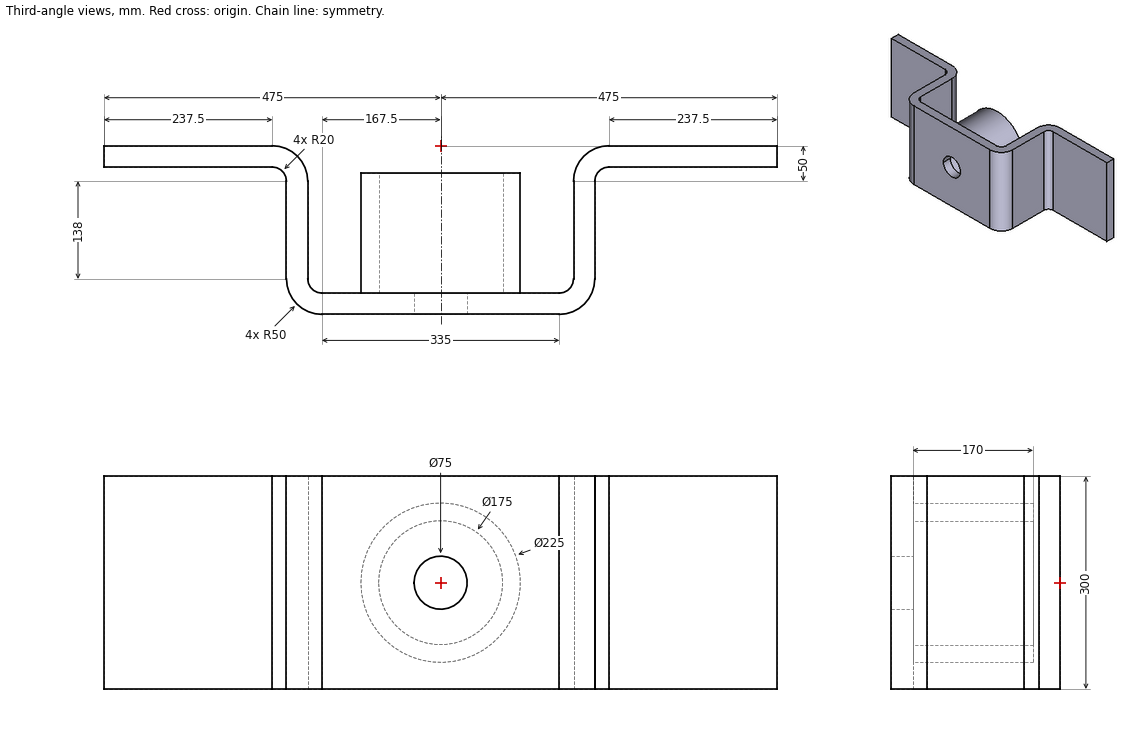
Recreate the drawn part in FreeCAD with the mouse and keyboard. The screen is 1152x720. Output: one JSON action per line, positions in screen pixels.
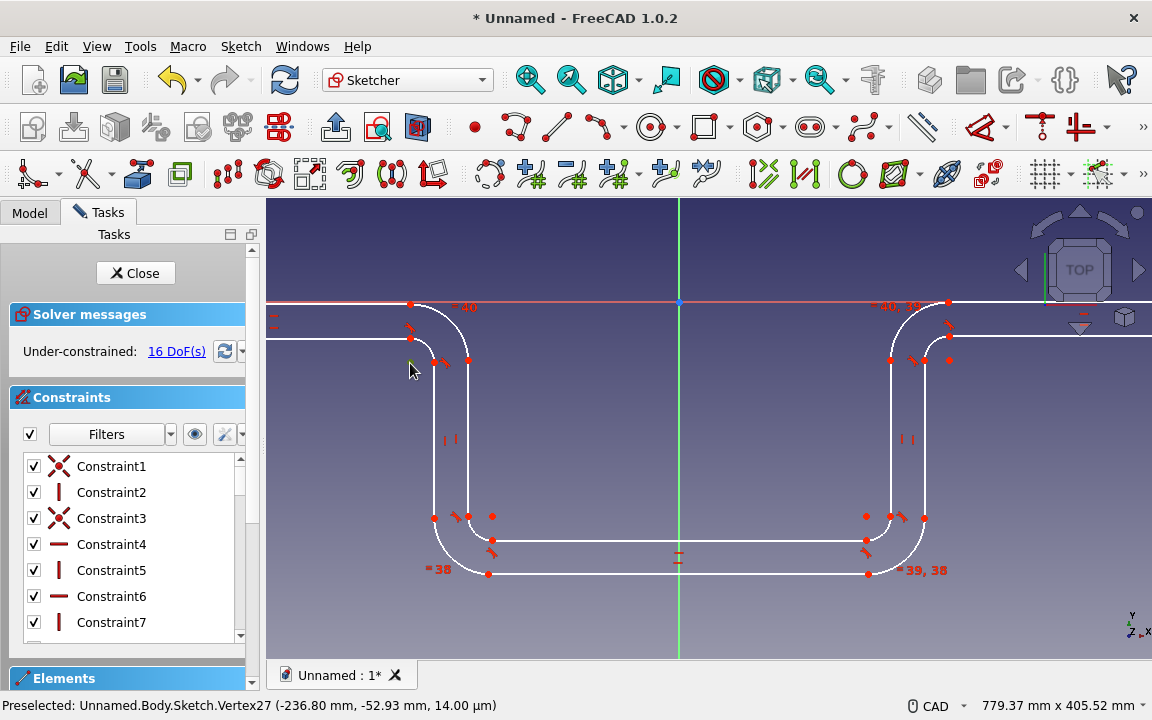
{"action": "left_click", "coordinate": [949, 361]}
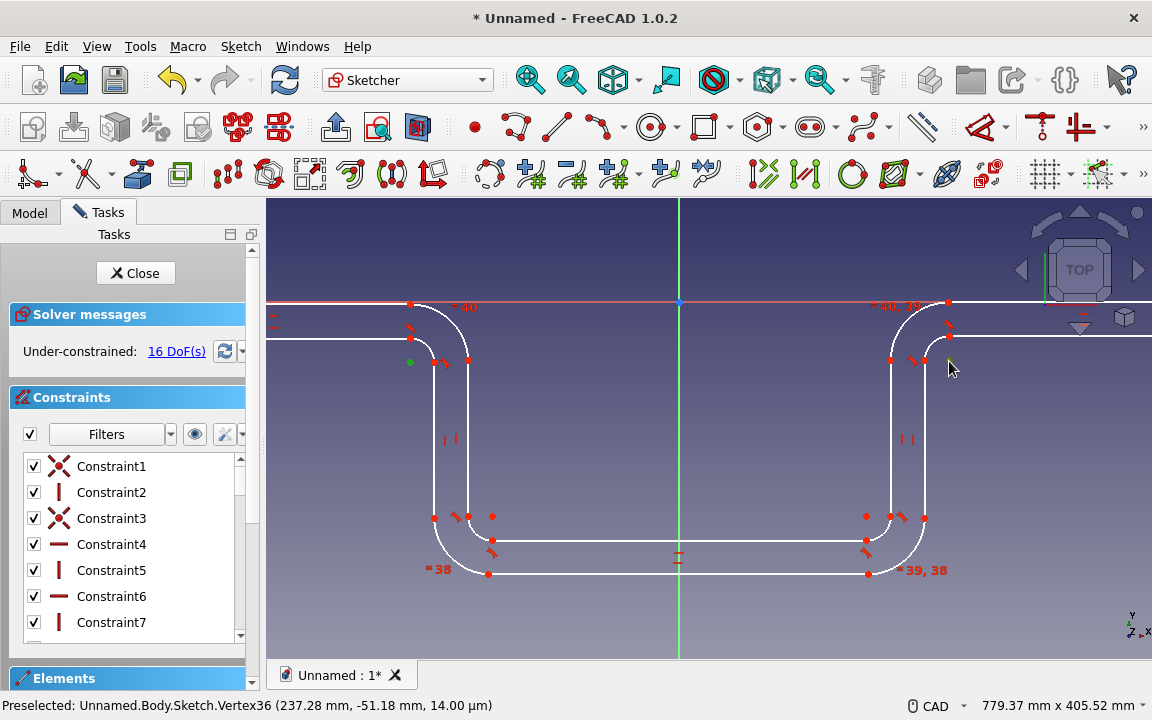
{"action": "left_click", "coordinate": [679, 486]}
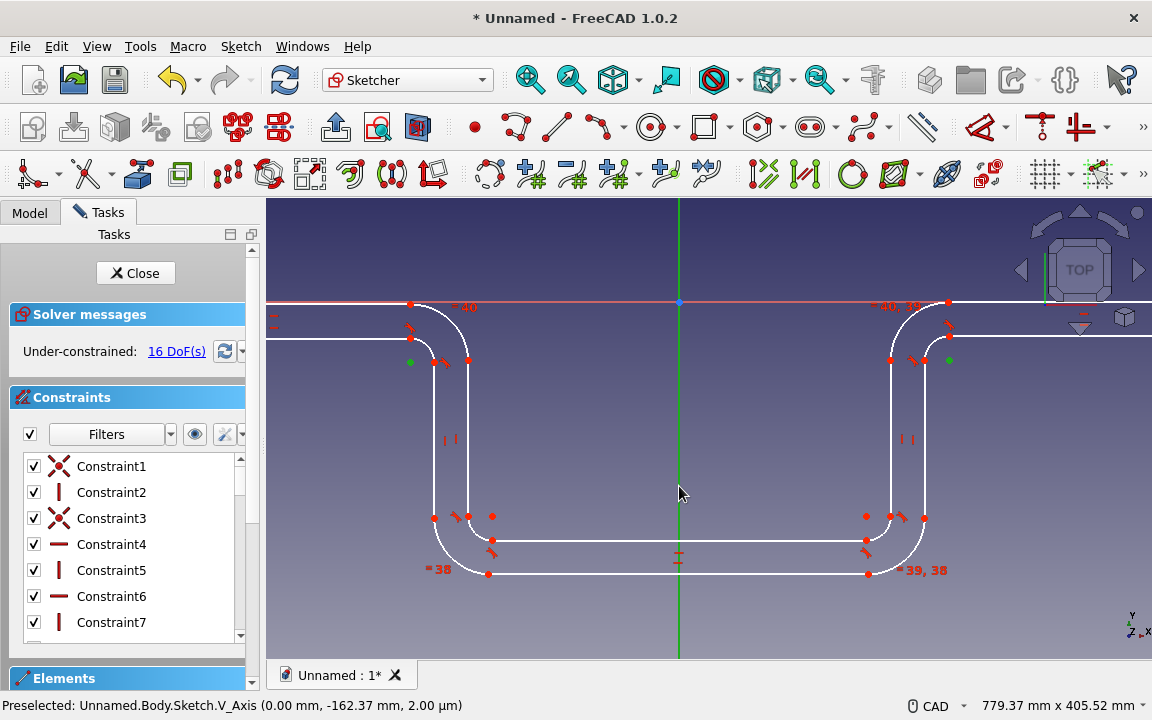
{"action": "key", "text": "s"}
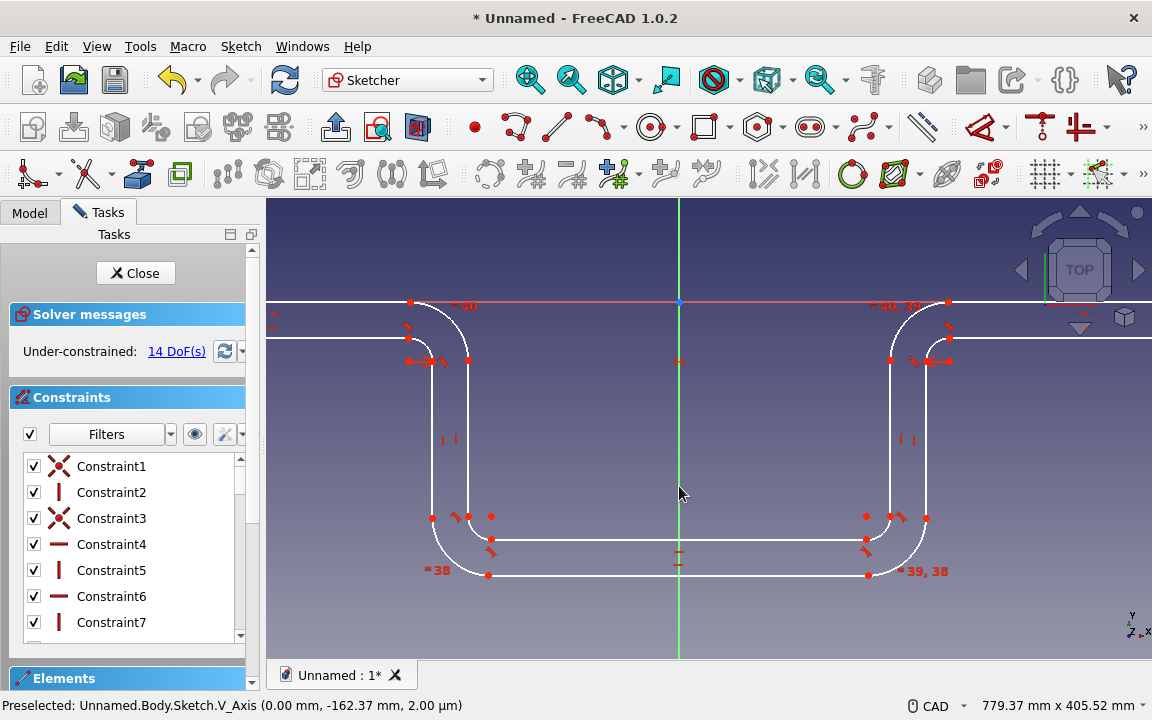
{"action": "key", "text": "d"}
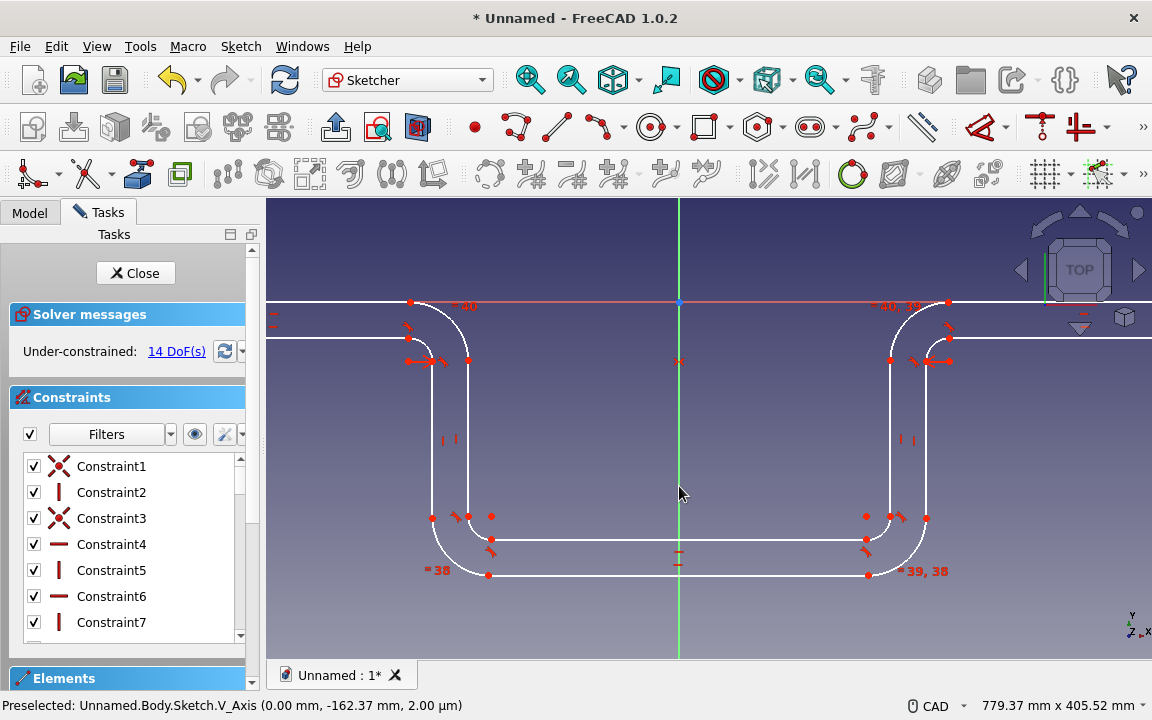
{"action": "scroll", "coordinate": [430, 351], "scroll_direction": "up", "scroll_amount": 3}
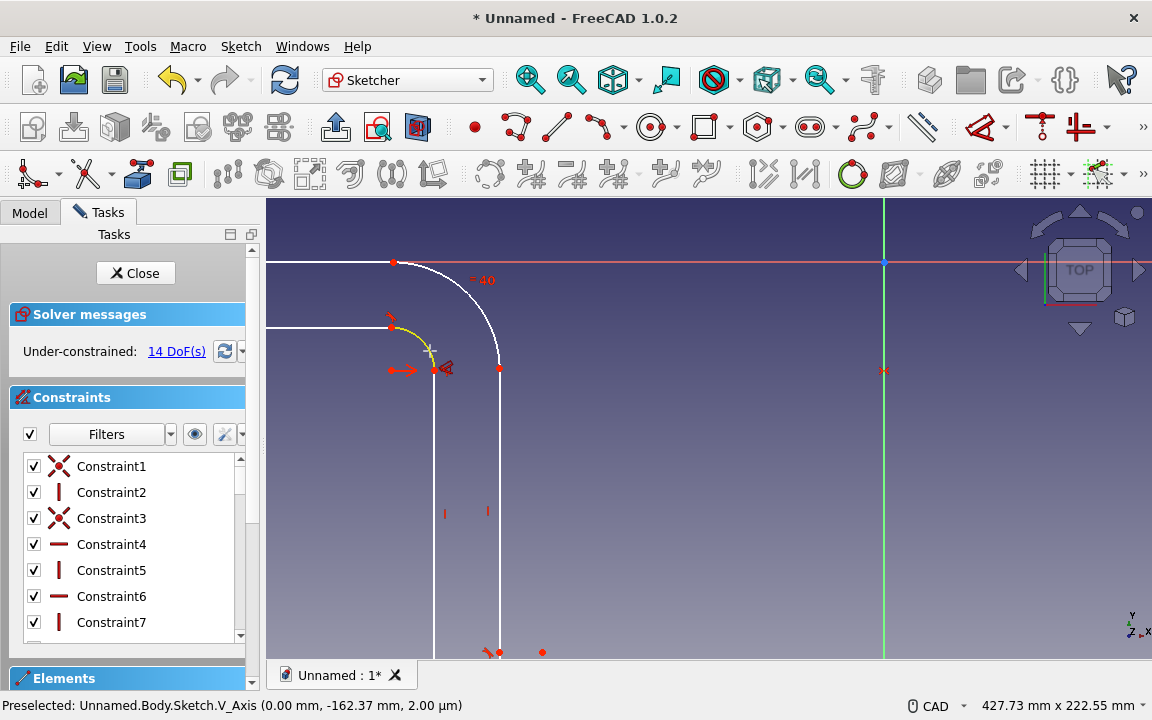
{"action": "left_click", "coordinate": [430, 351]}
{"action": "left_click", "coordinate": [459, 337]}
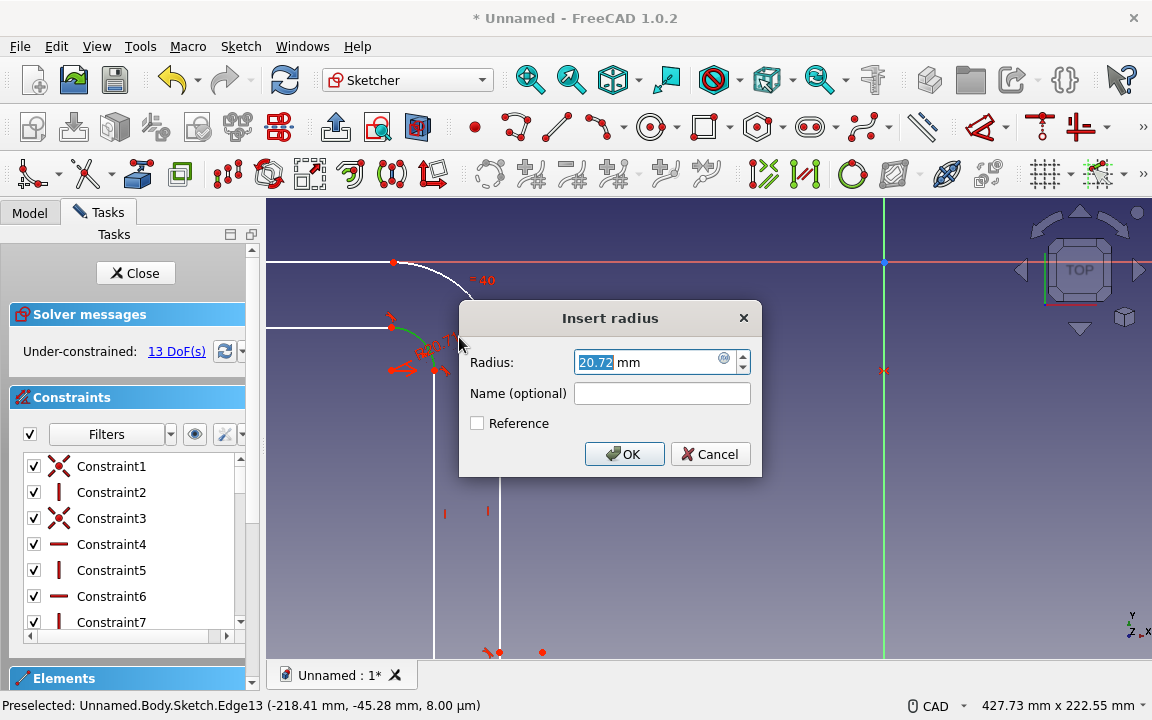
{"action": "type", "text": "20"}
{"action": "key", "text": "Return"}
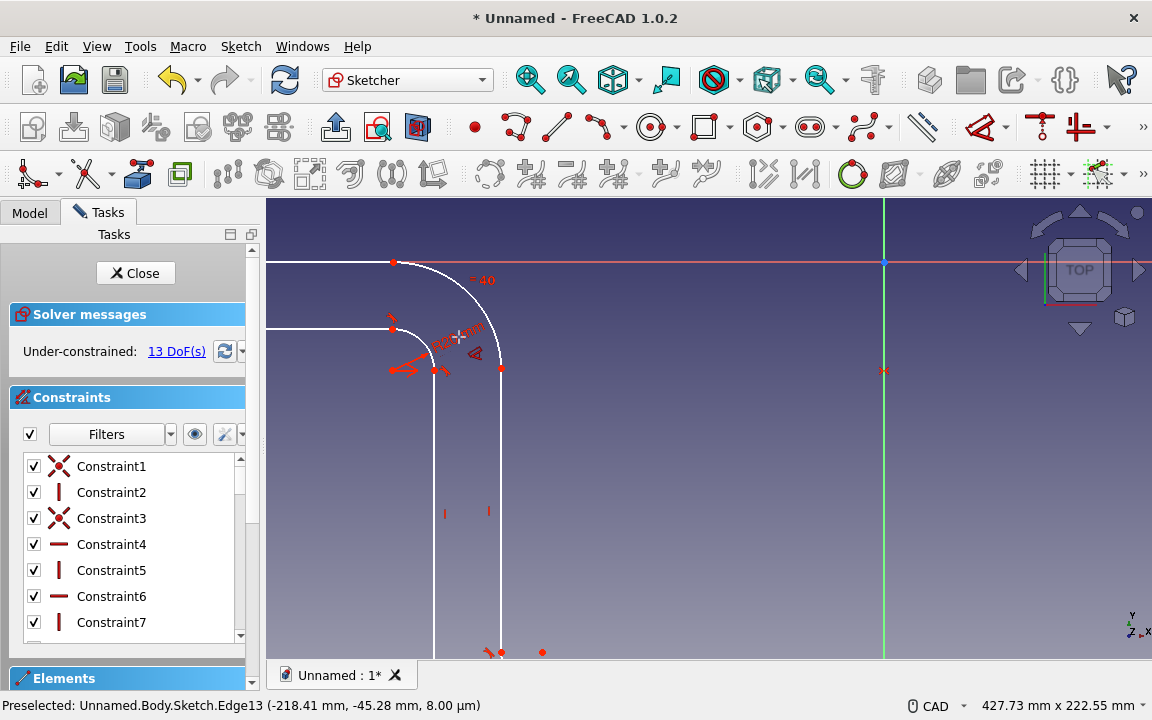
{"action": "scroll", "coordinate": [561, 402], "scroll_direction": "down", "scroll_amount": 7}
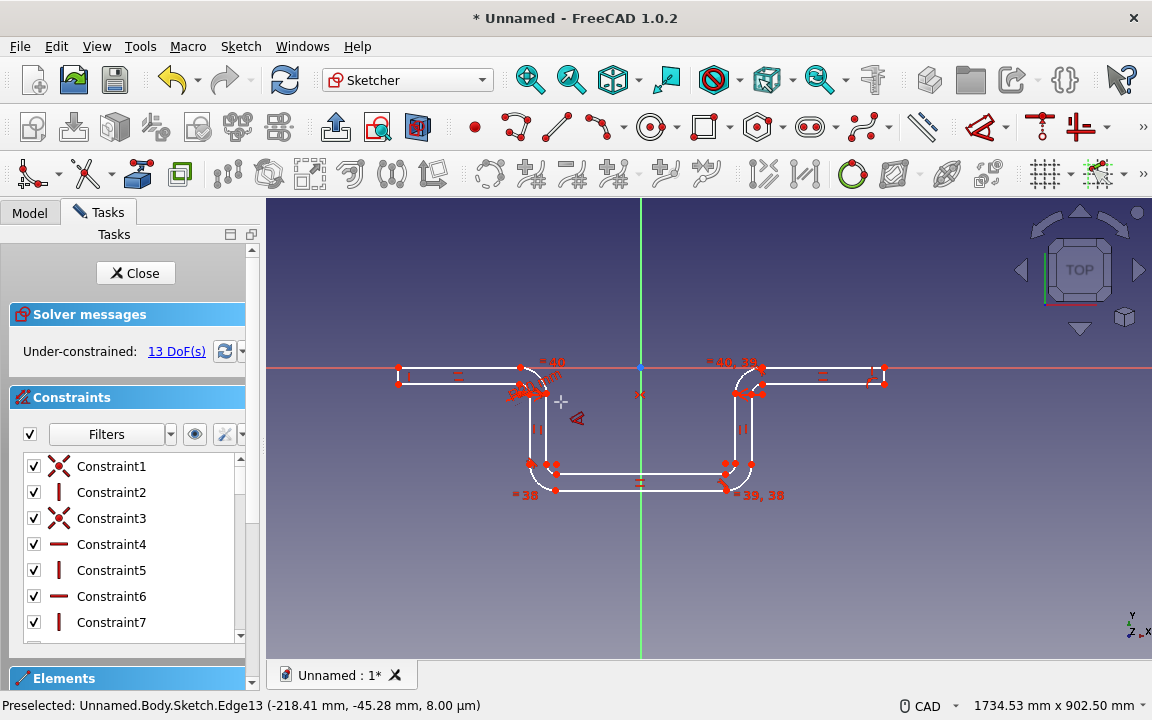
{"action": "scroll", "coordinate": [533, 476], "scroll_direction": "up", "scroll_amount": 3}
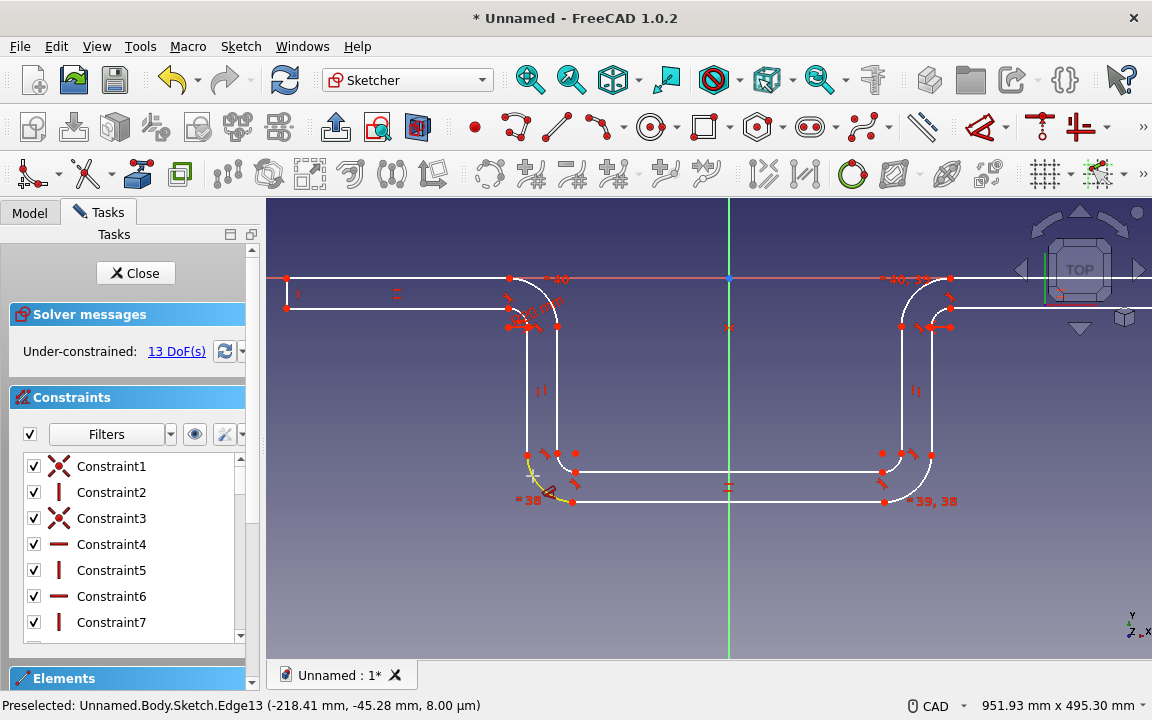
{"action": "left_click", "coordinate": [533, 476]}
{"action": "left_click", "coordinate": [505, 491]}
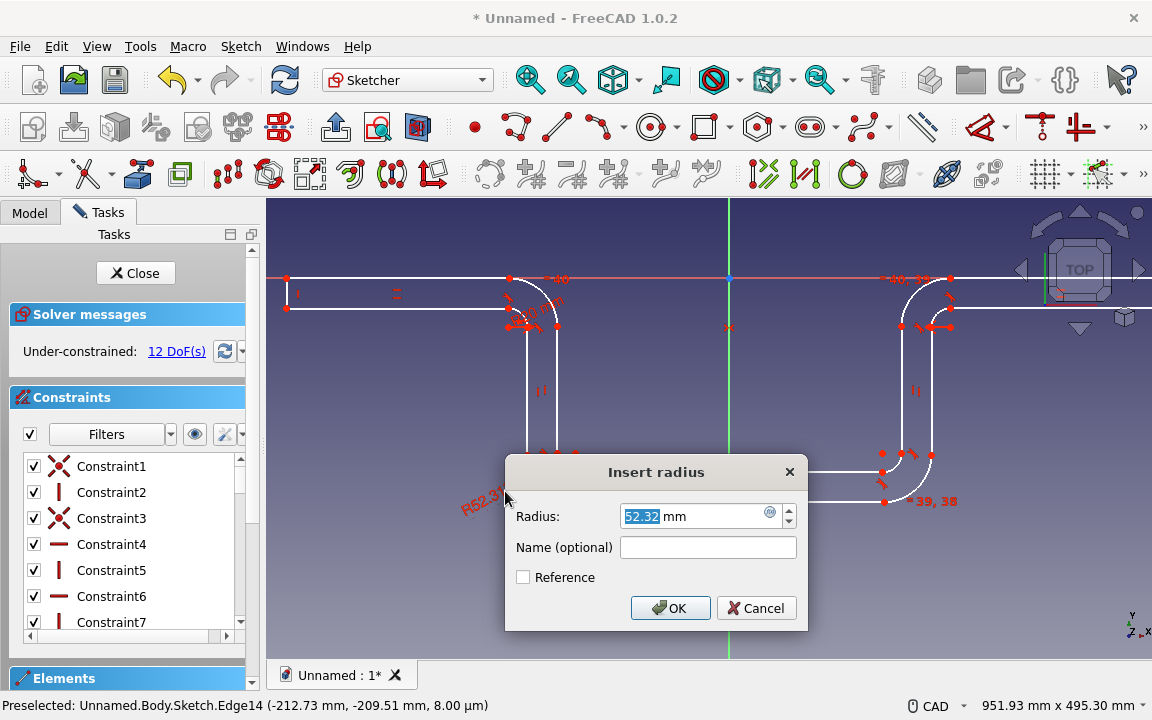
{"action": "type", "text": "50"}
{"action": "key", "text": "Return"}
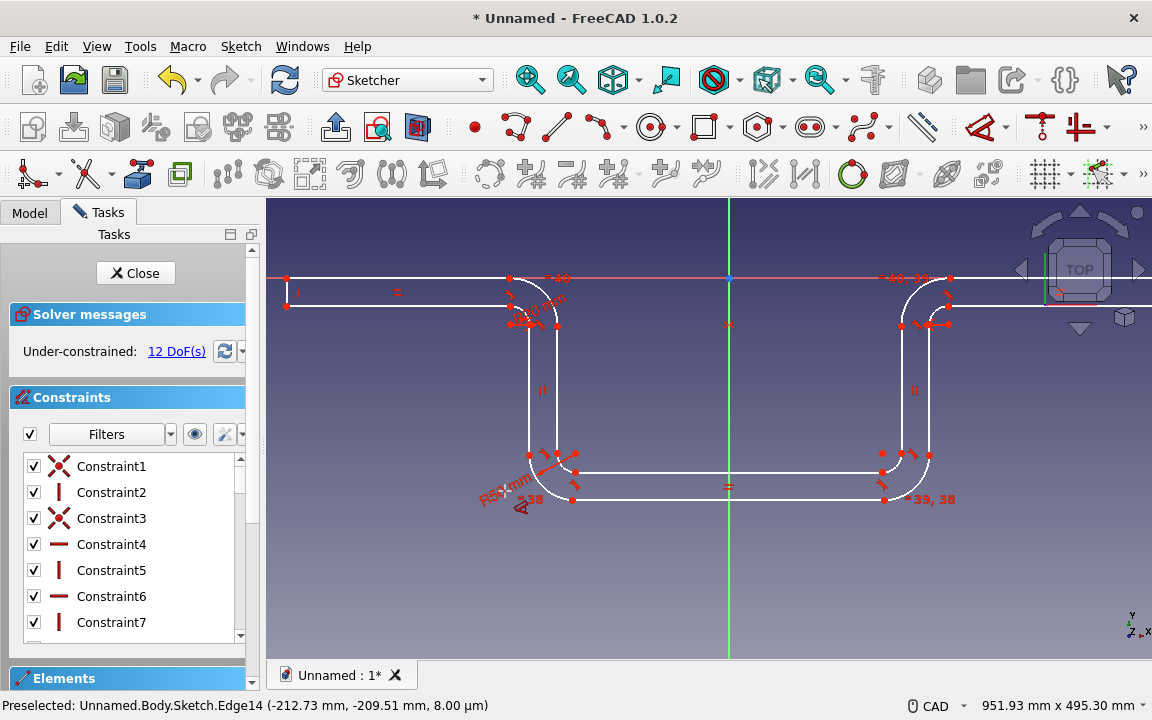
{"action": "left_click", "coordinate": [529, 364]}
{"action": "left_click", "coordinate": [495, 390]}